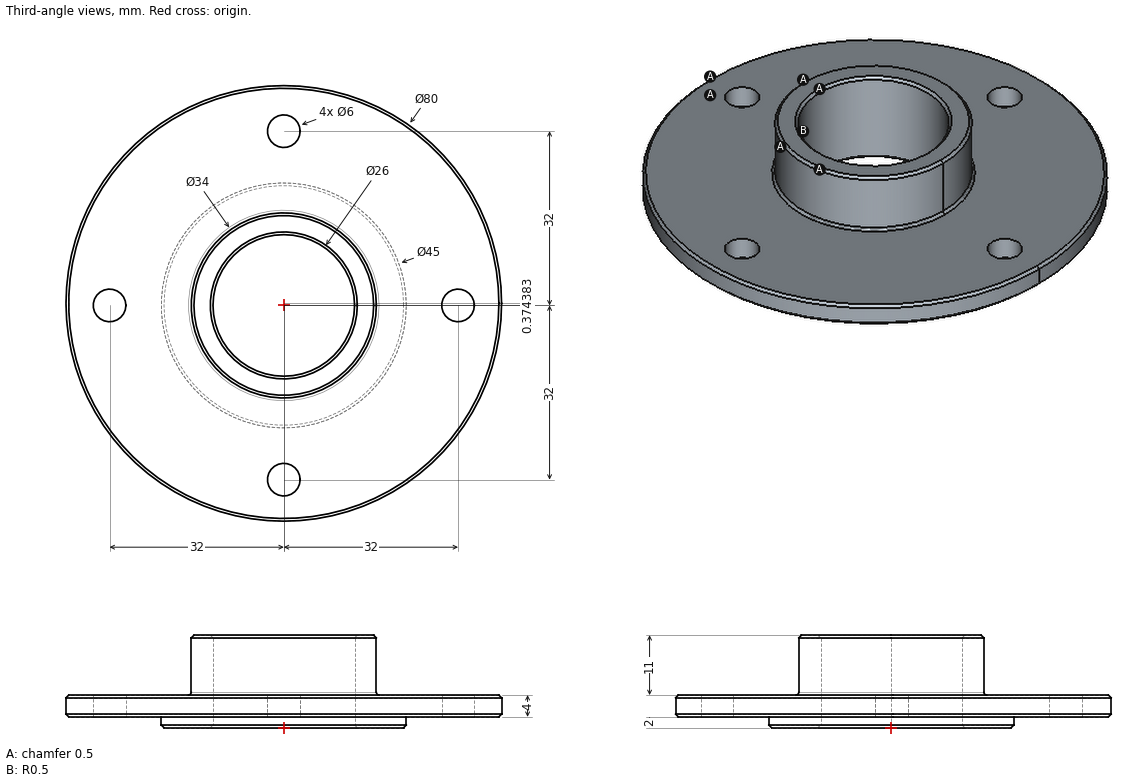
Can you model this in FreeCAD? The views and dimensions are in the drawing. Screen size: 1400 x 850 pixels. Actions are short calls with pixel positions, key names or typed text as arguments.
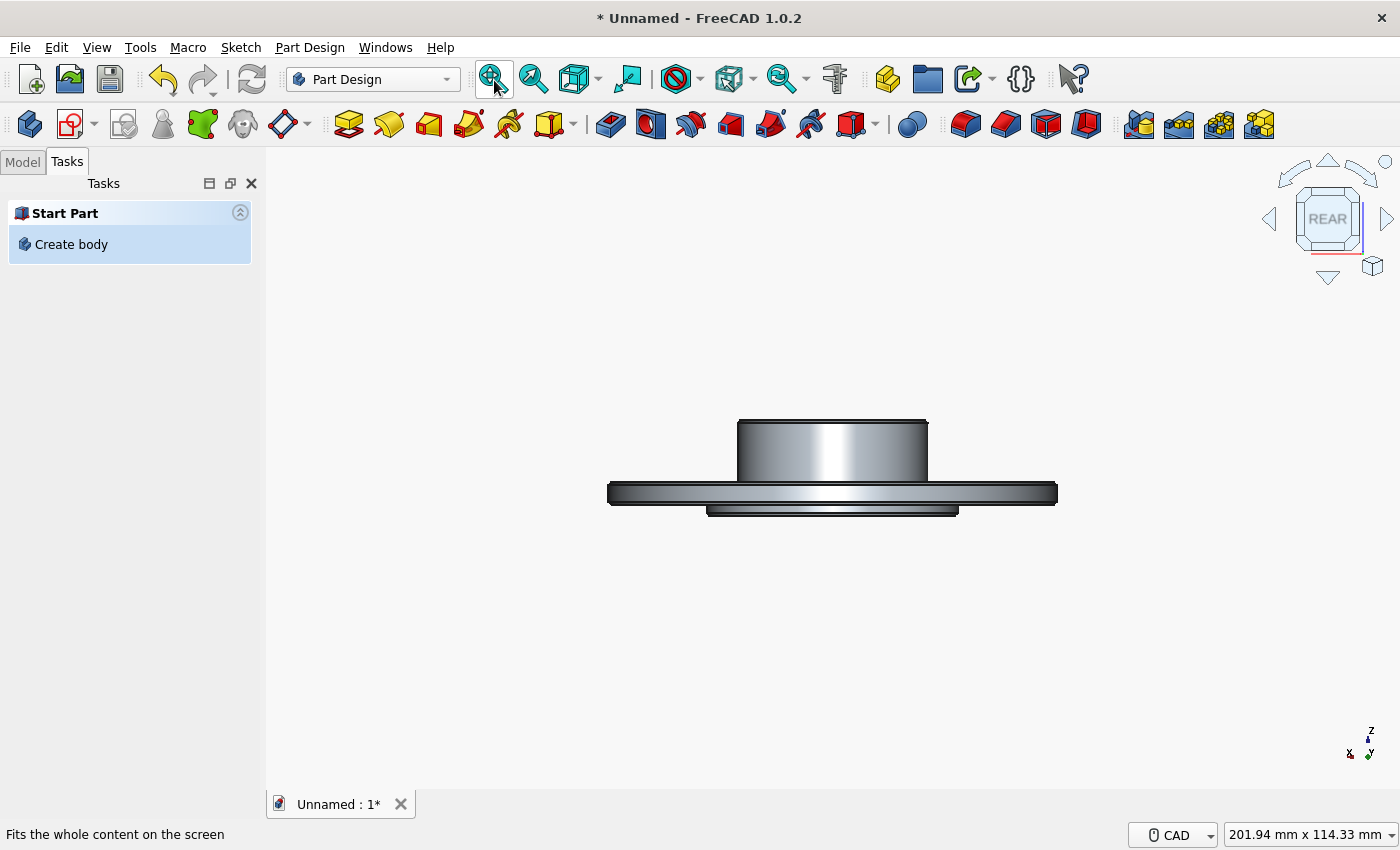
click(494, 80)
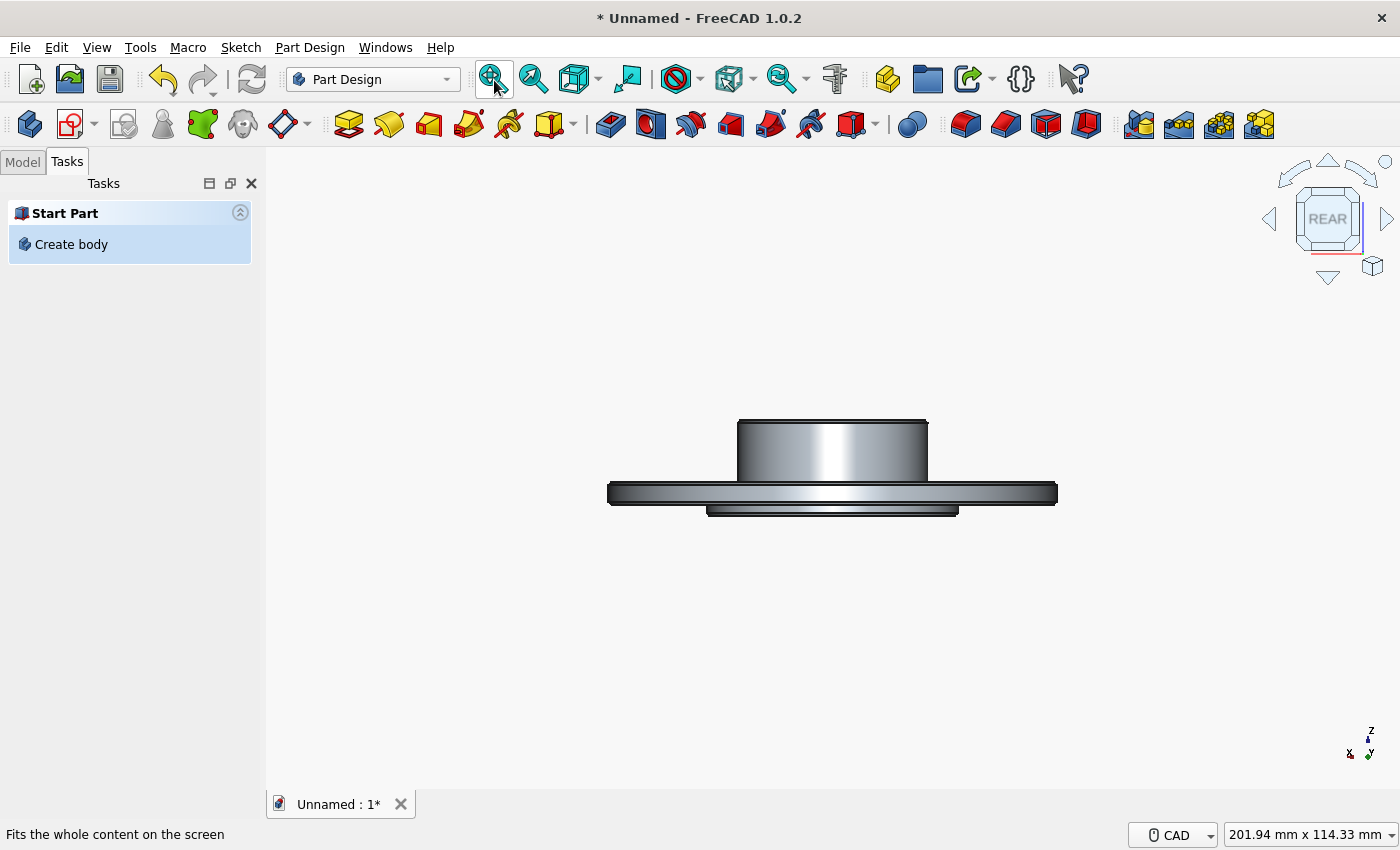
key(6)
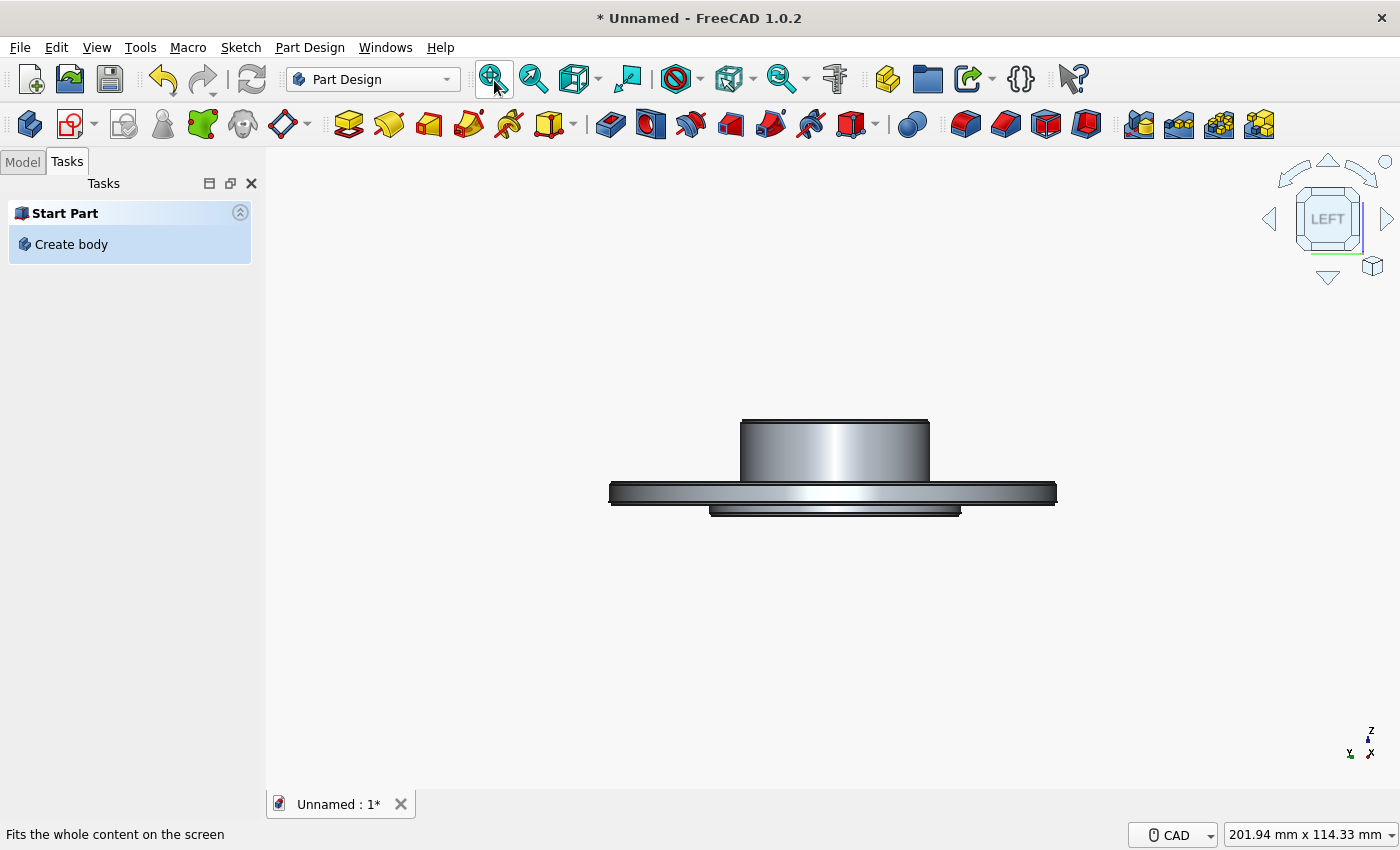
click(494, 80)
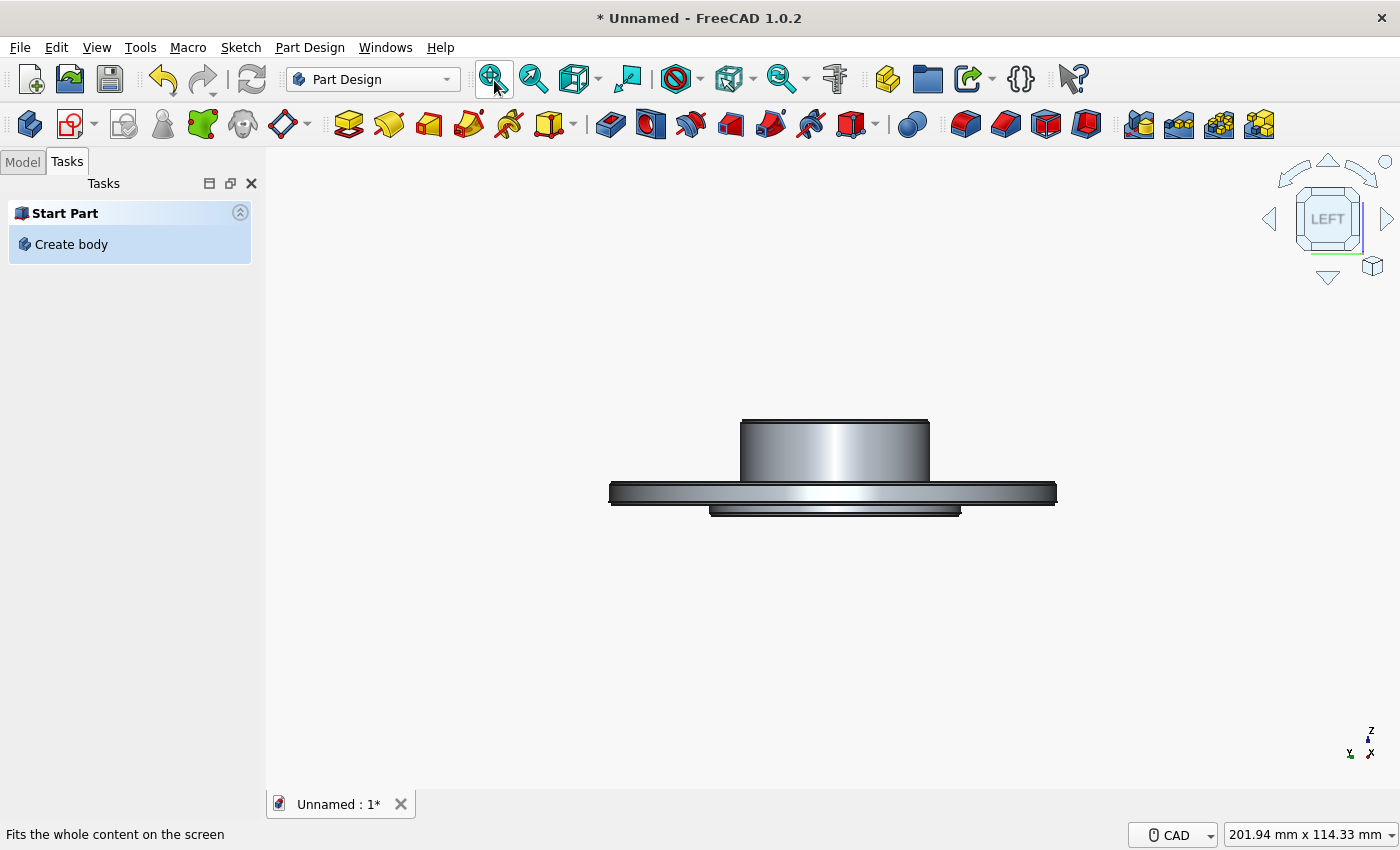
key(v)
key(3)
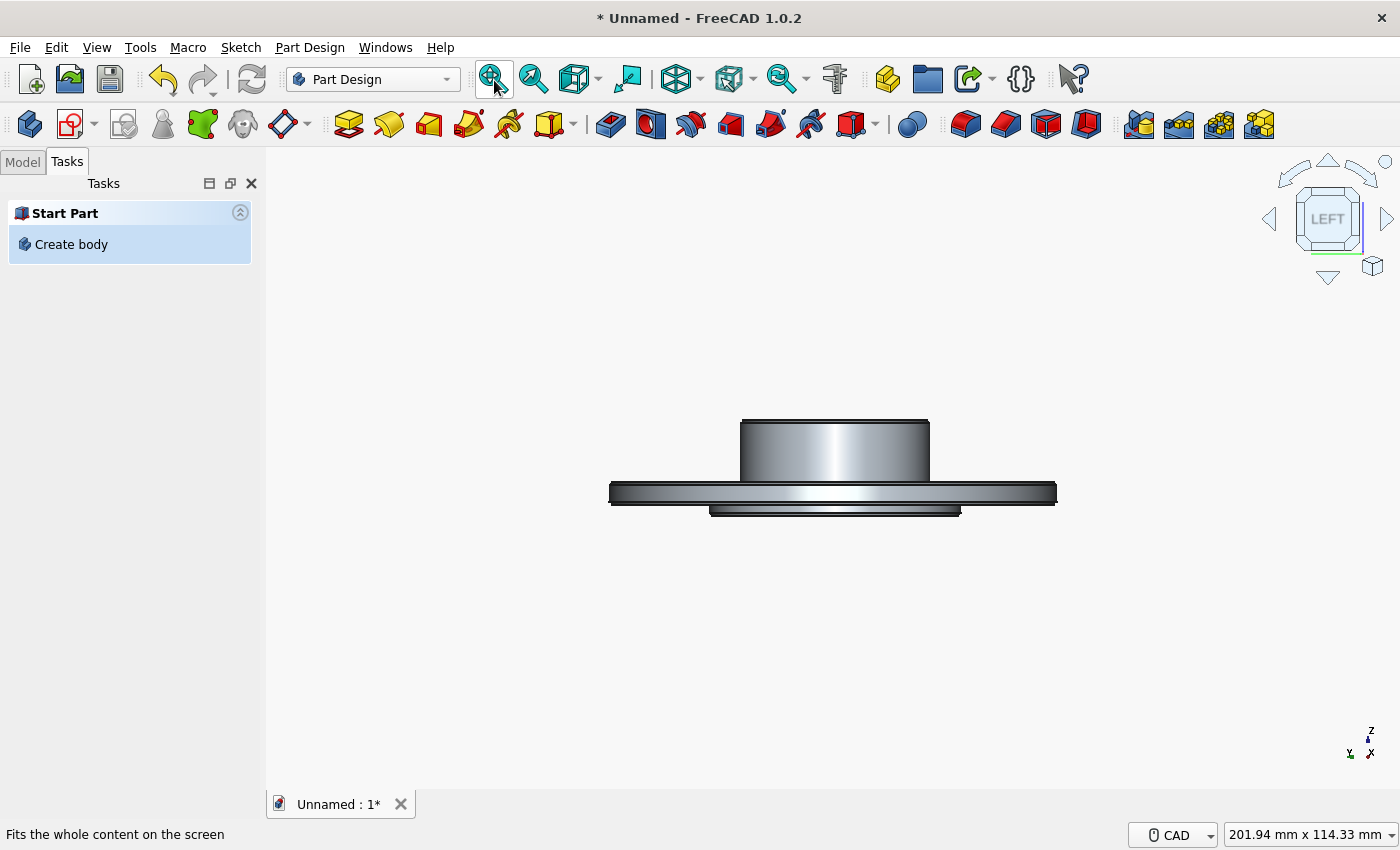
key(0)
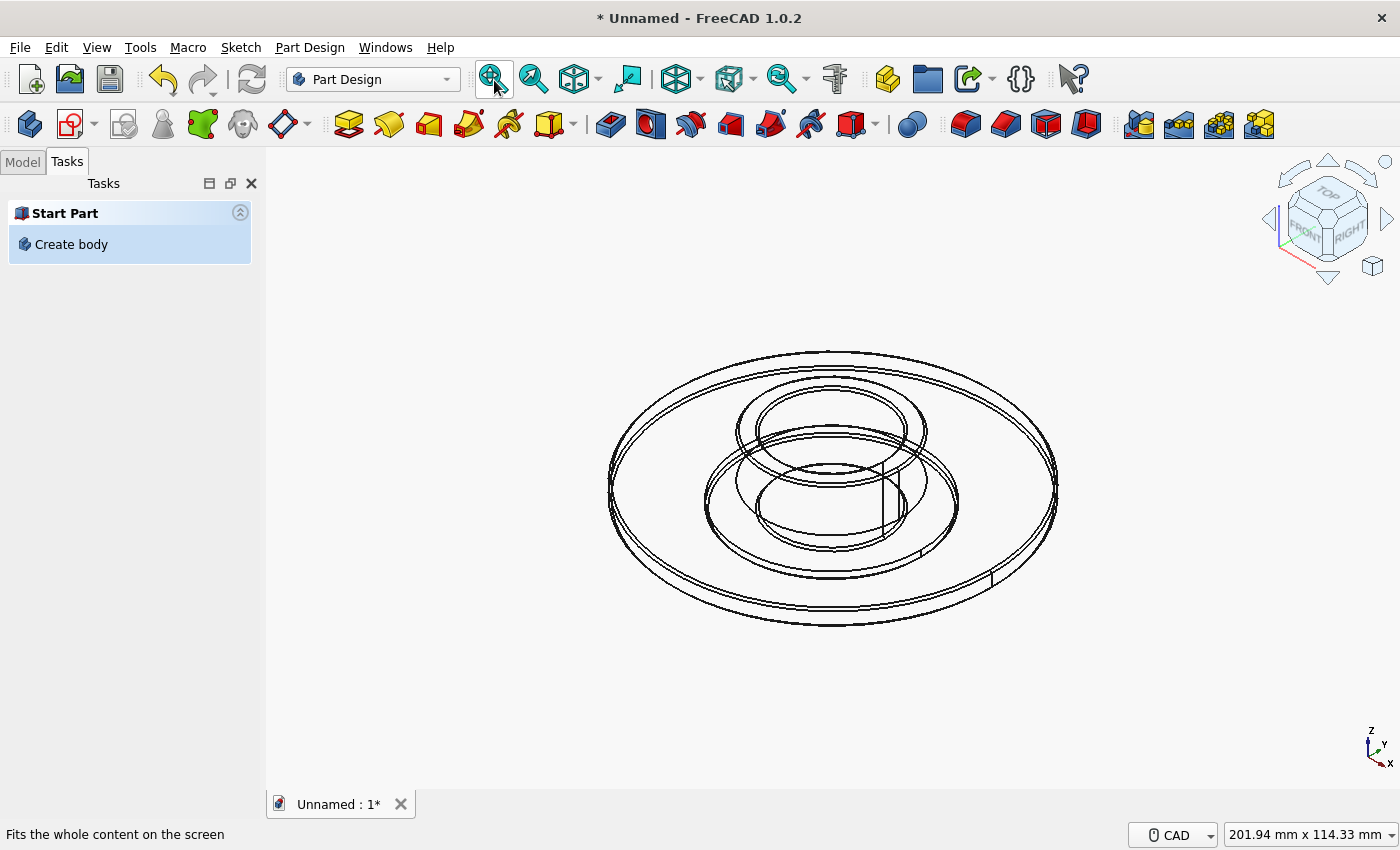
click(817, 425)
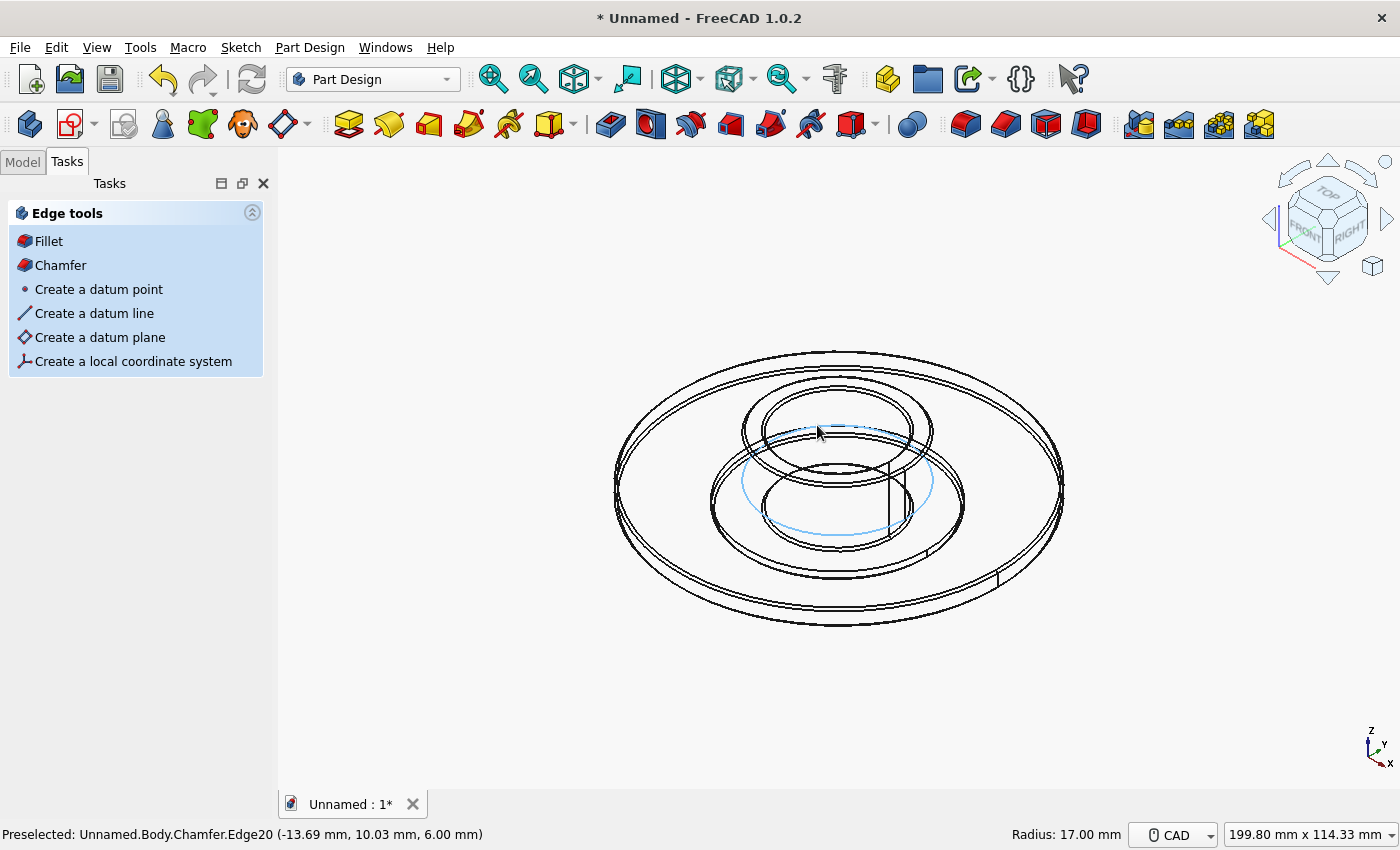
key(v)
key(1)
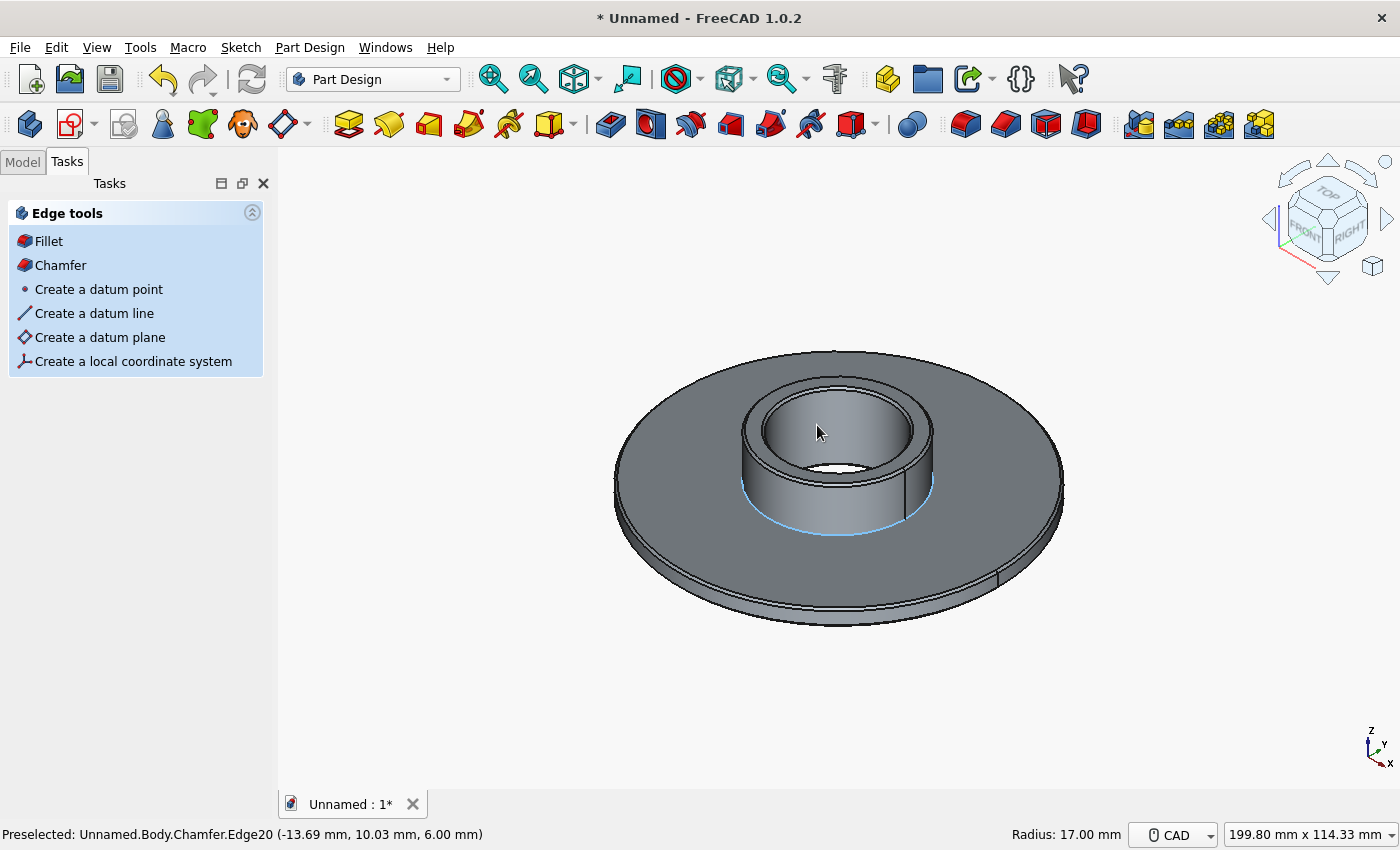
click(966, 124)